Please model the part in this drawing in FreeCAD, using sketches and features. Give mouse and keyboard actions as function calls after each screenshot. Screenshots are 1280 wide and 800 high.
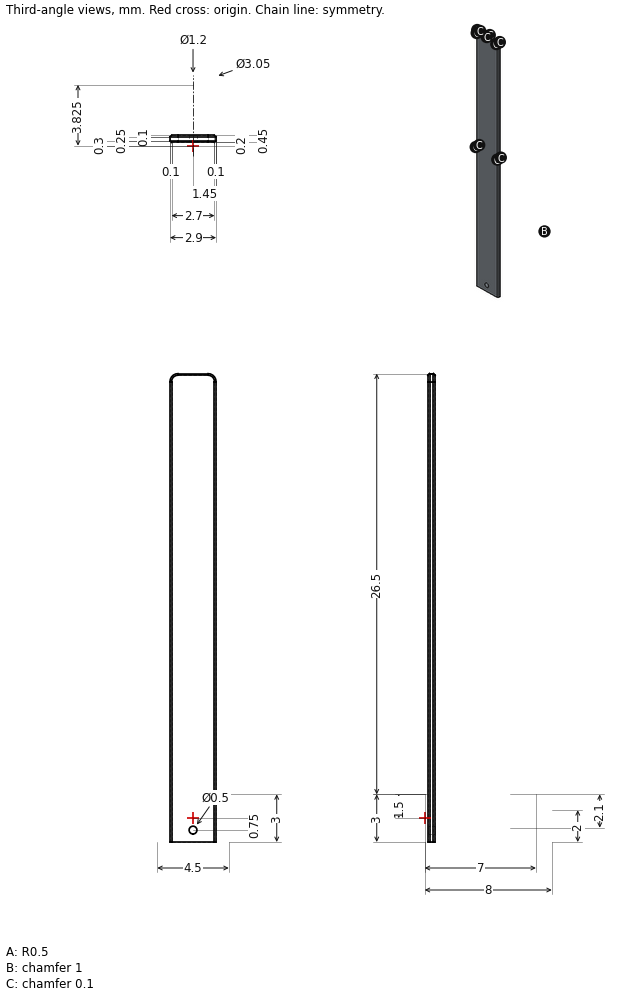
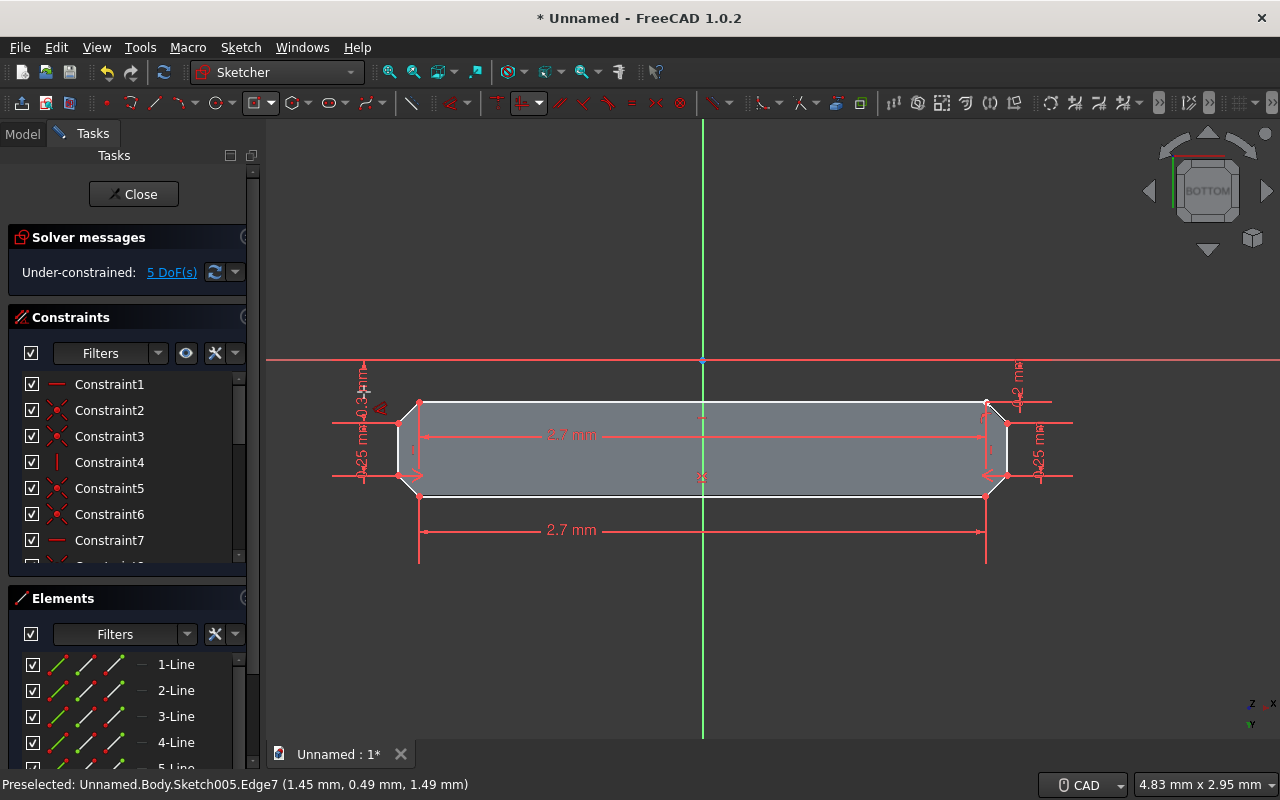
scroll(411, 410, up, 4)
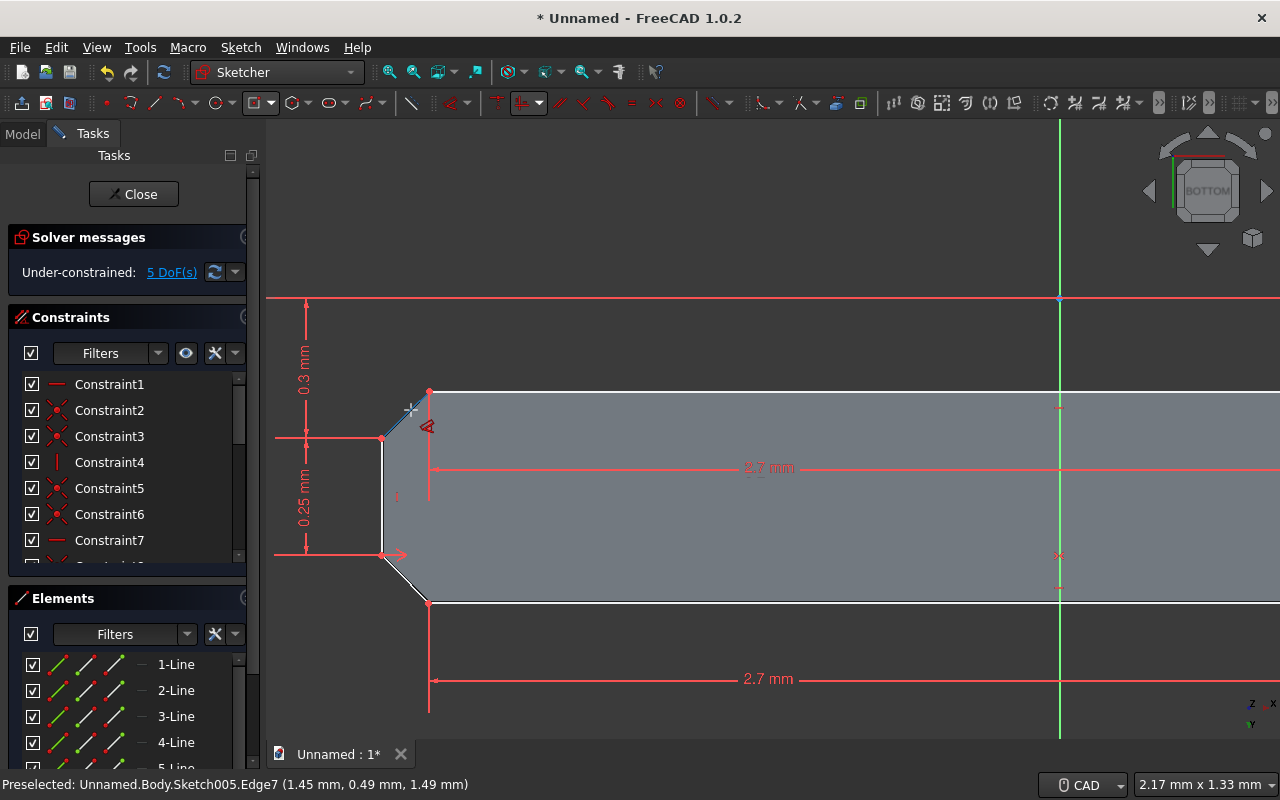
click(410, 410)
click(406, 358)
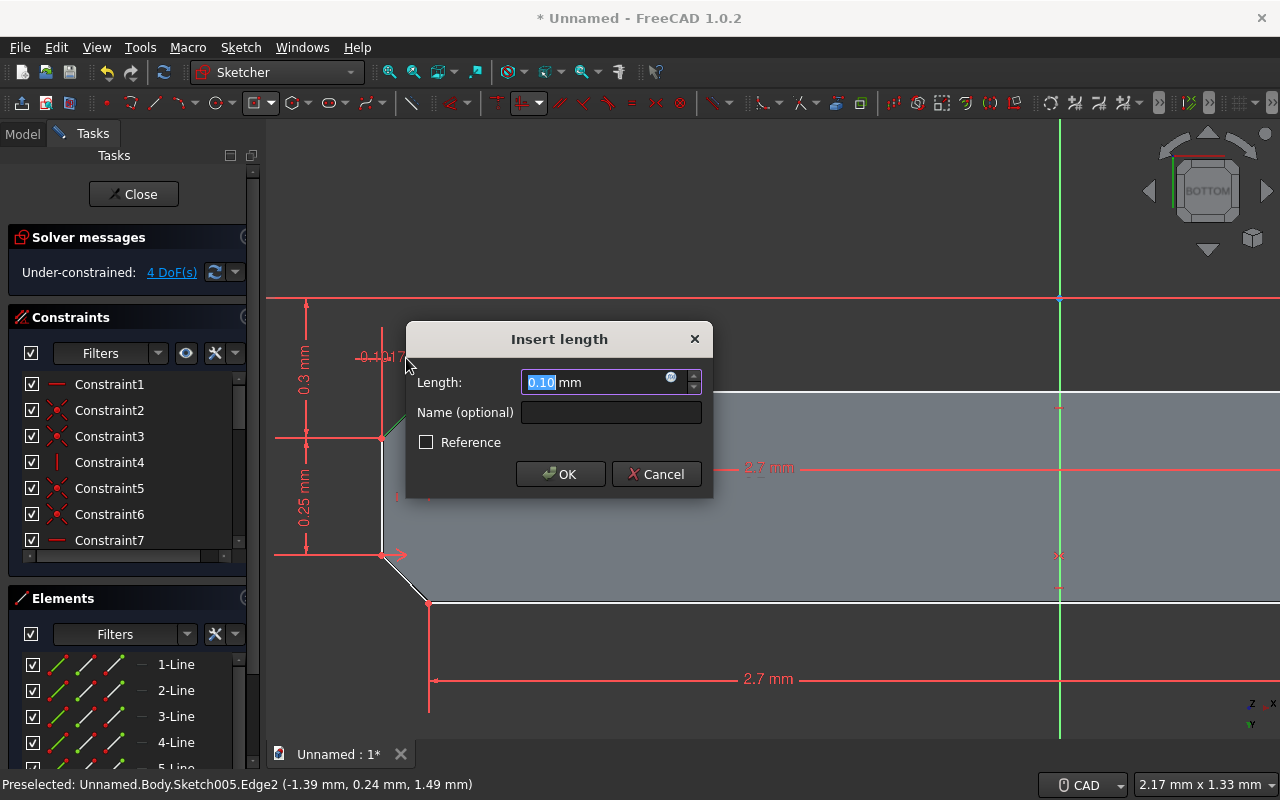
text(0.1)
key(Return)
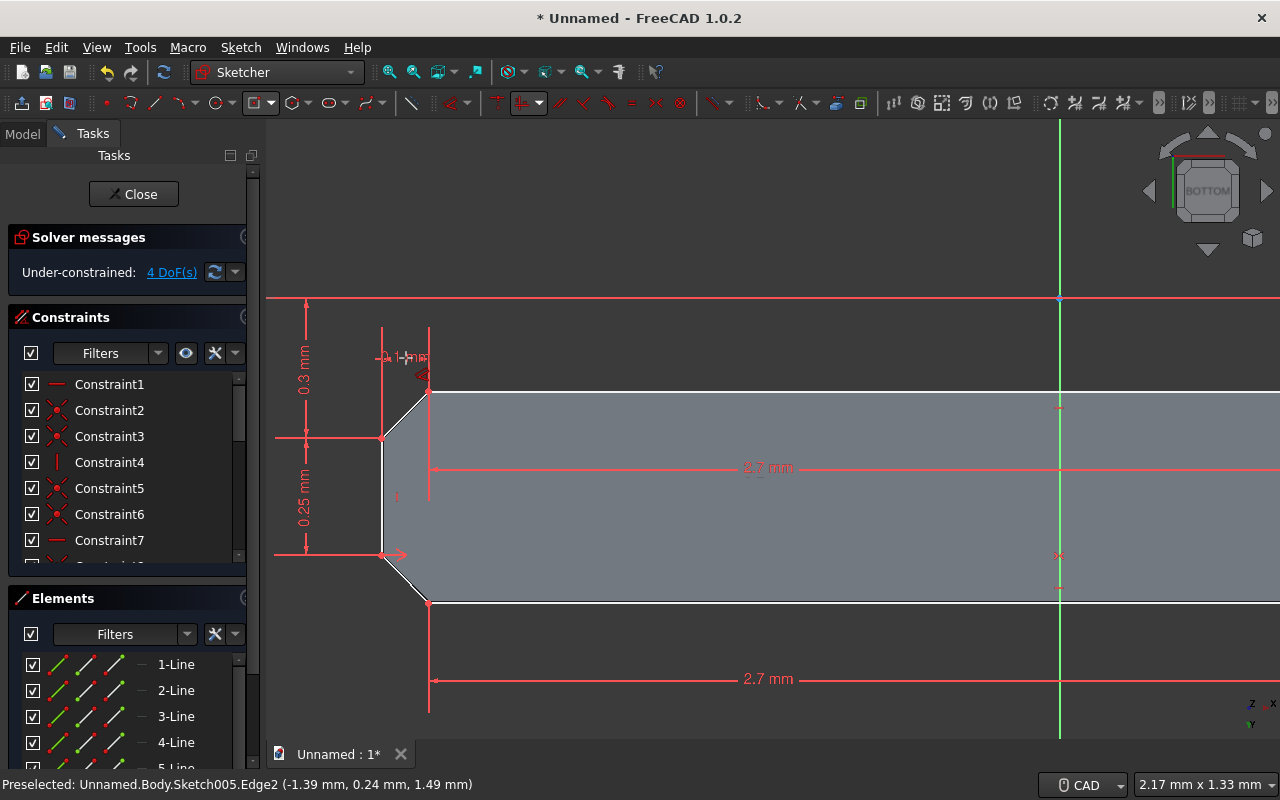
click(396, 570)
click(405, 637)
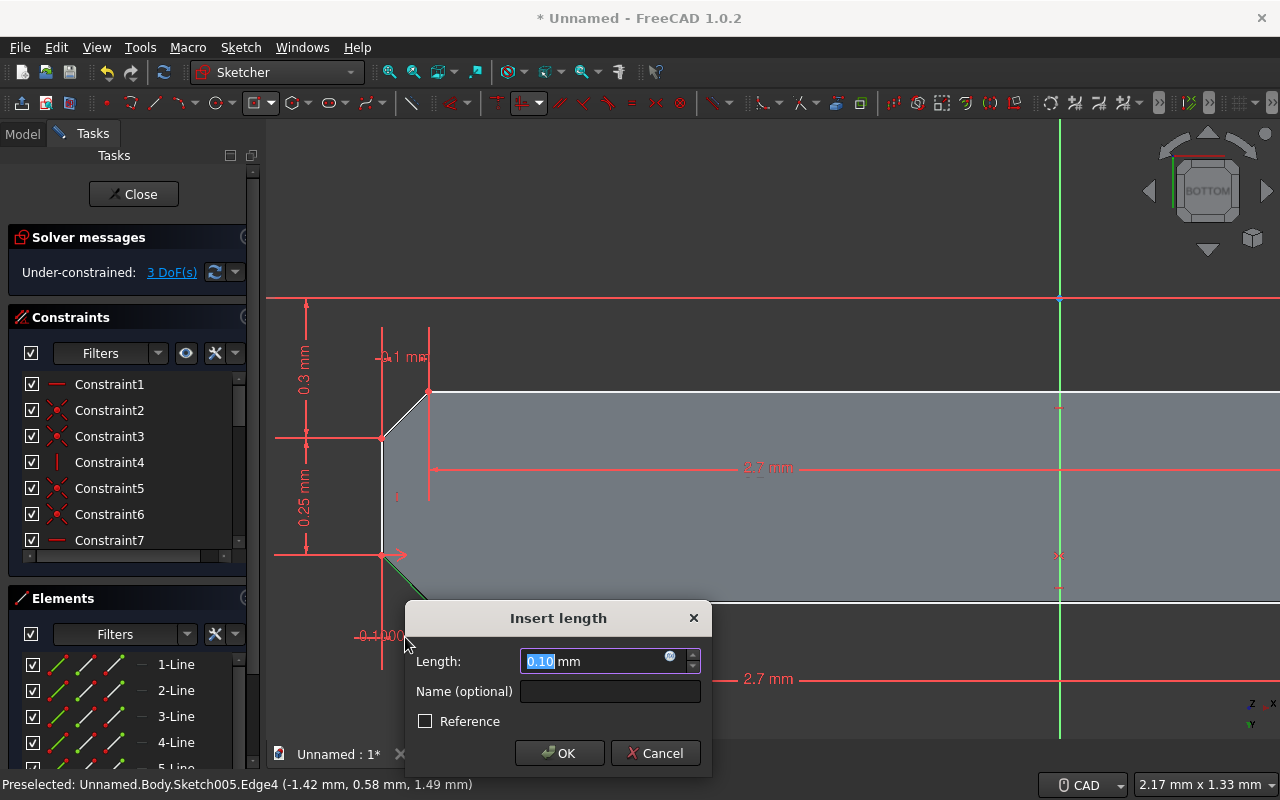
text(0.1)
key(Return)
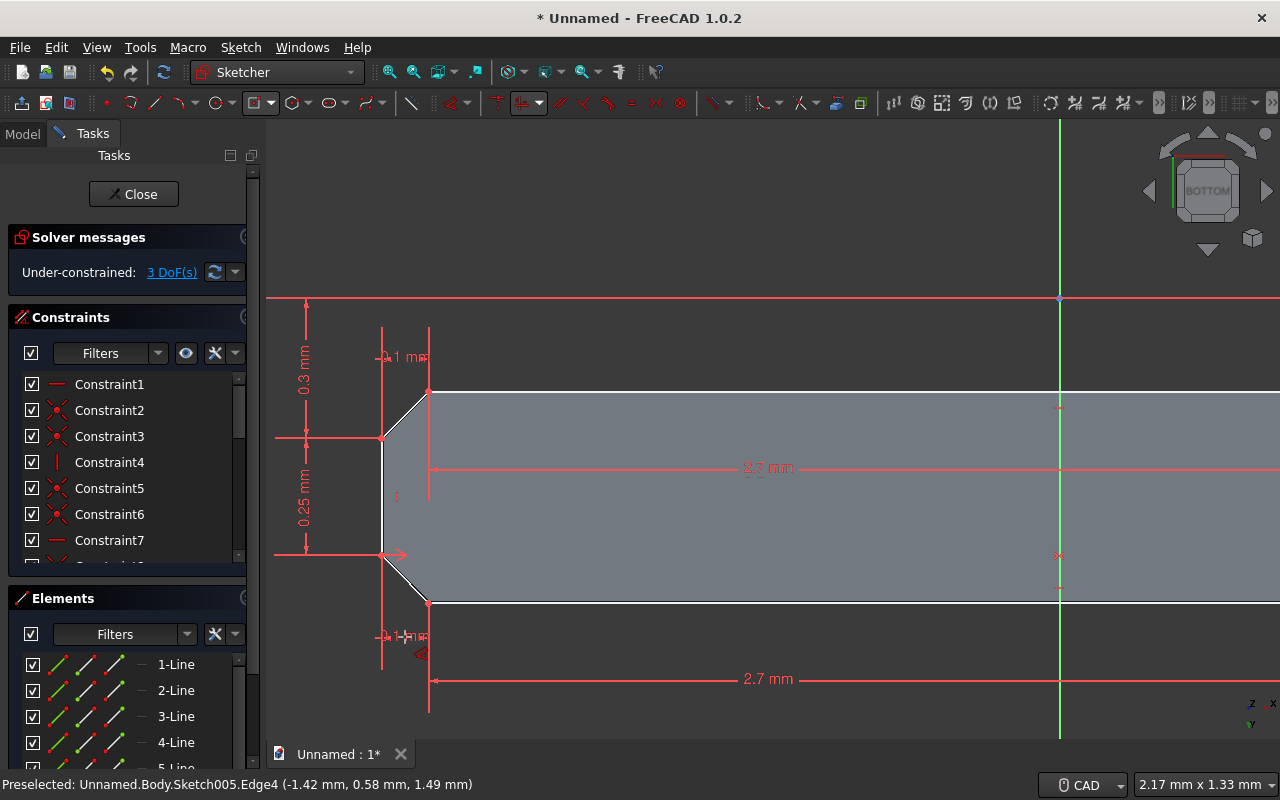
click(396, 570)
click(348, 579)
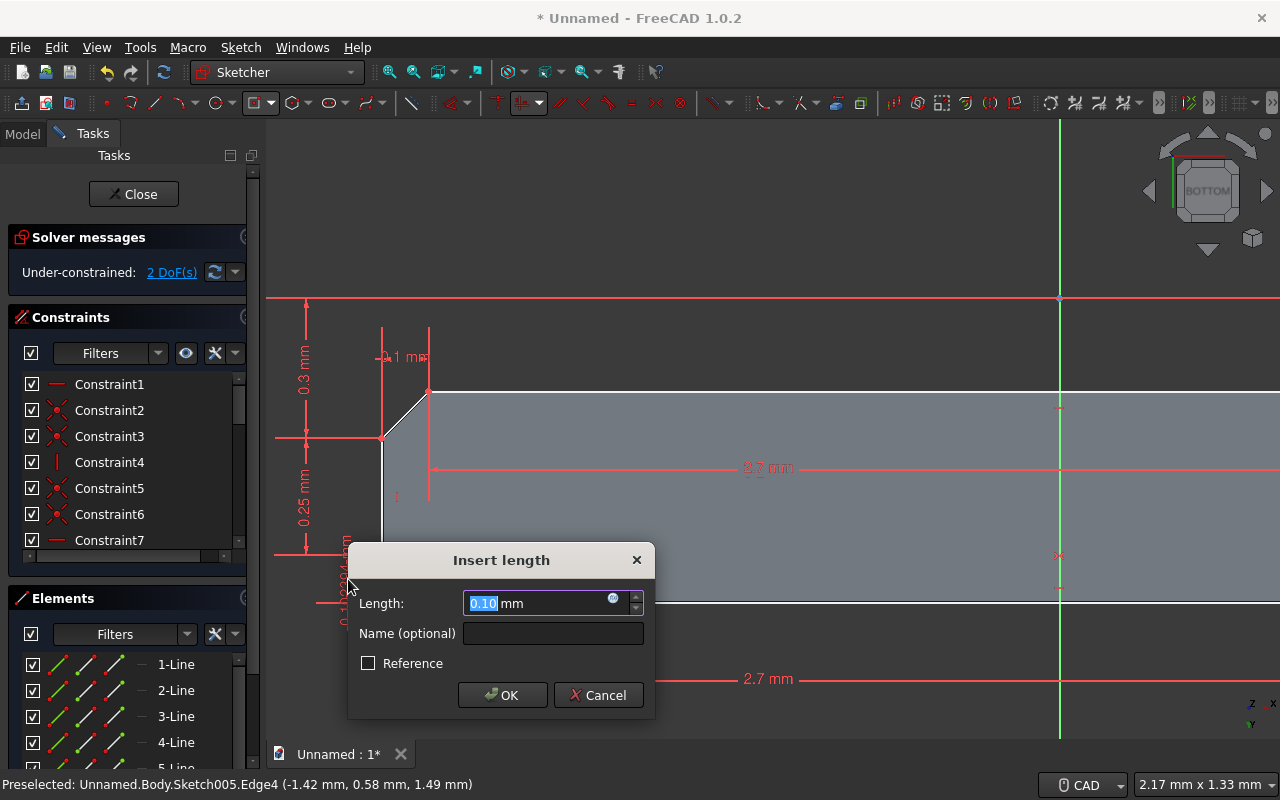
text(0.1)
key(Return)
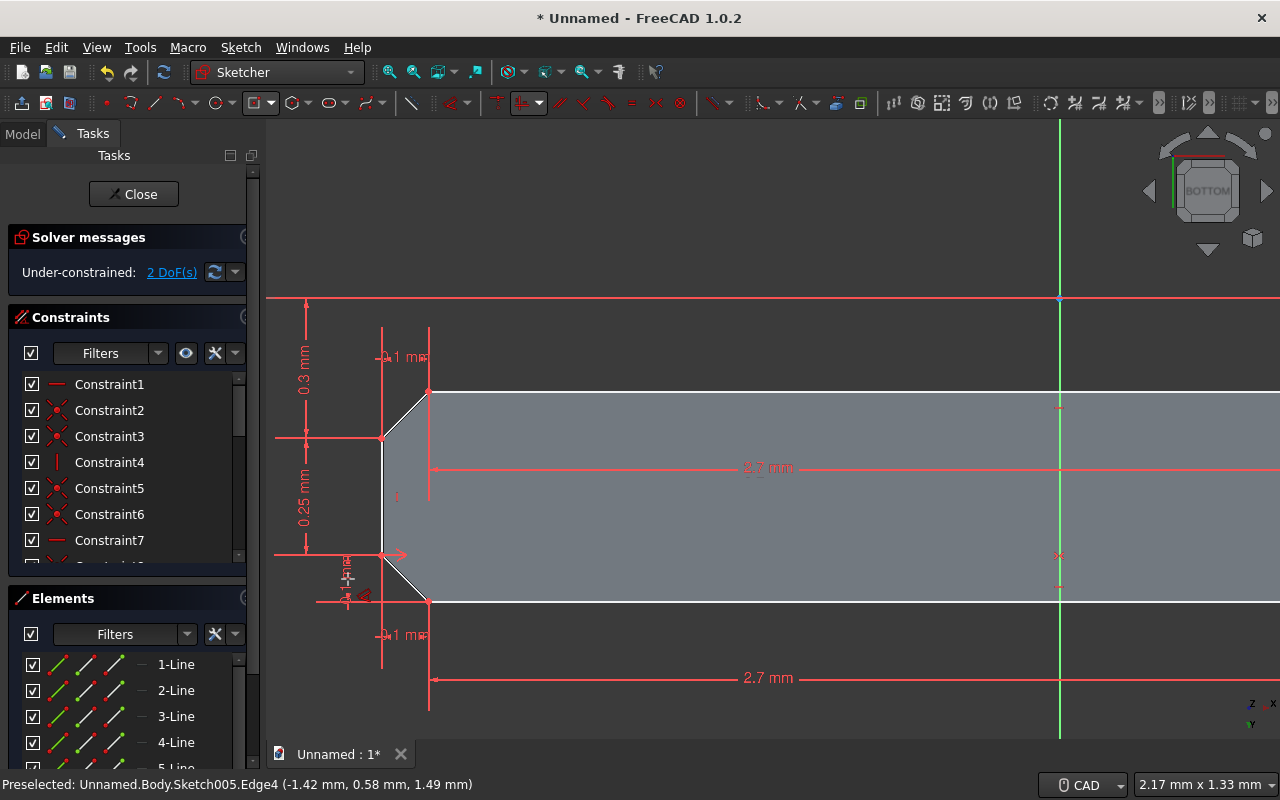
scroll(415, 412, down, 4)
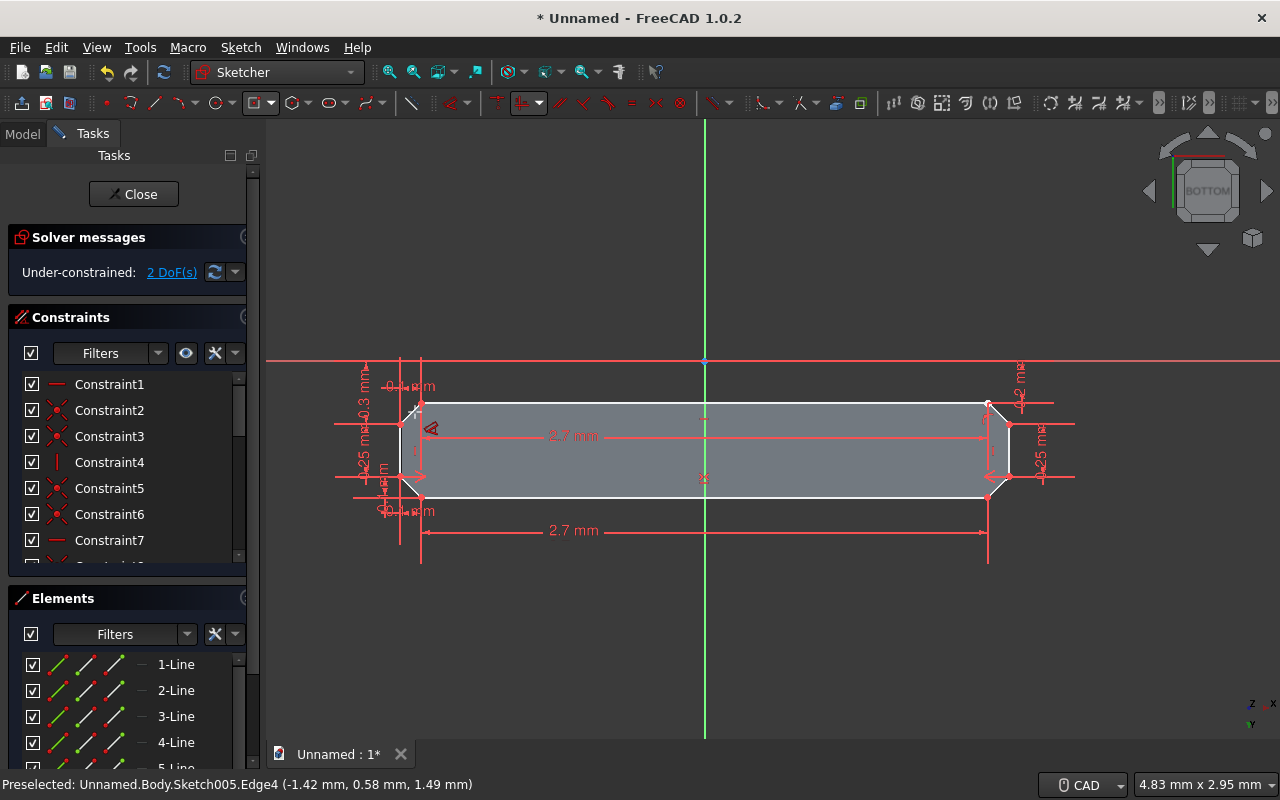
scroll(994, 491, up, 4)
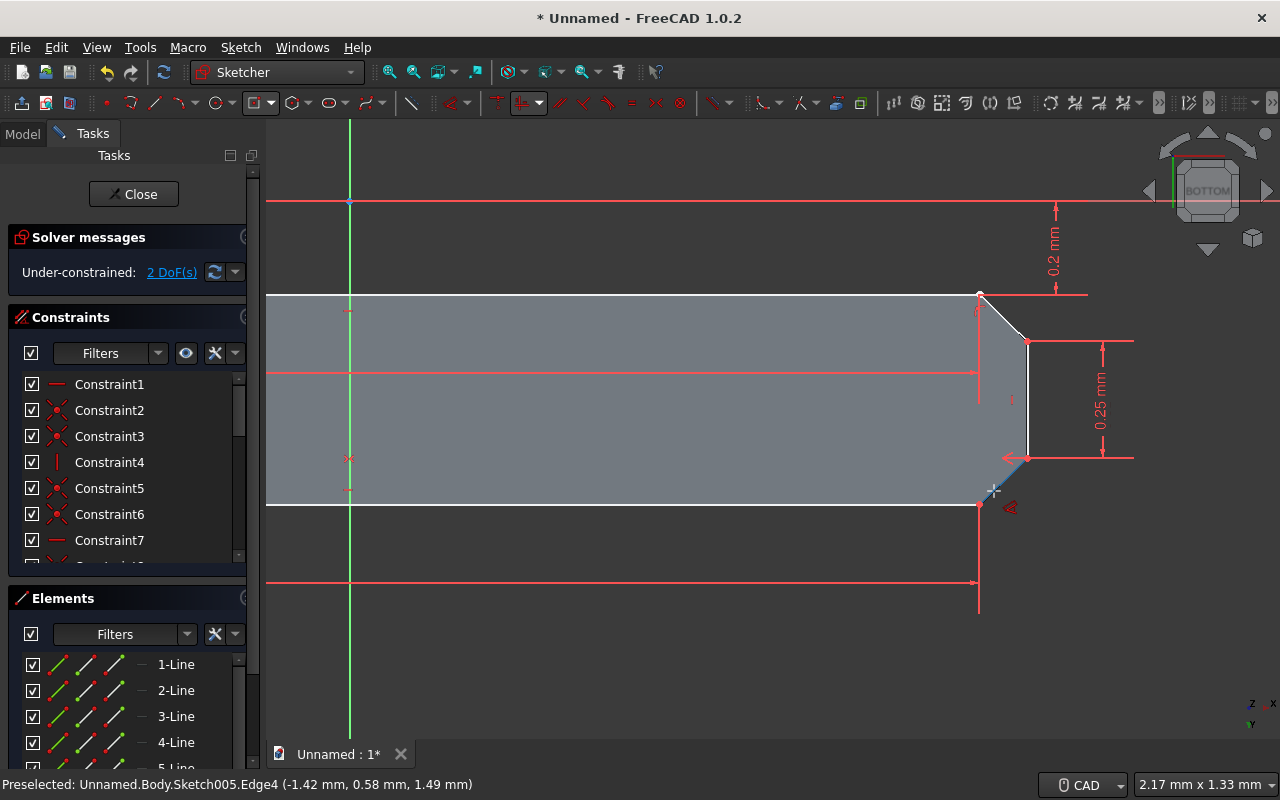
click(994, 491)
click(1004, 539)